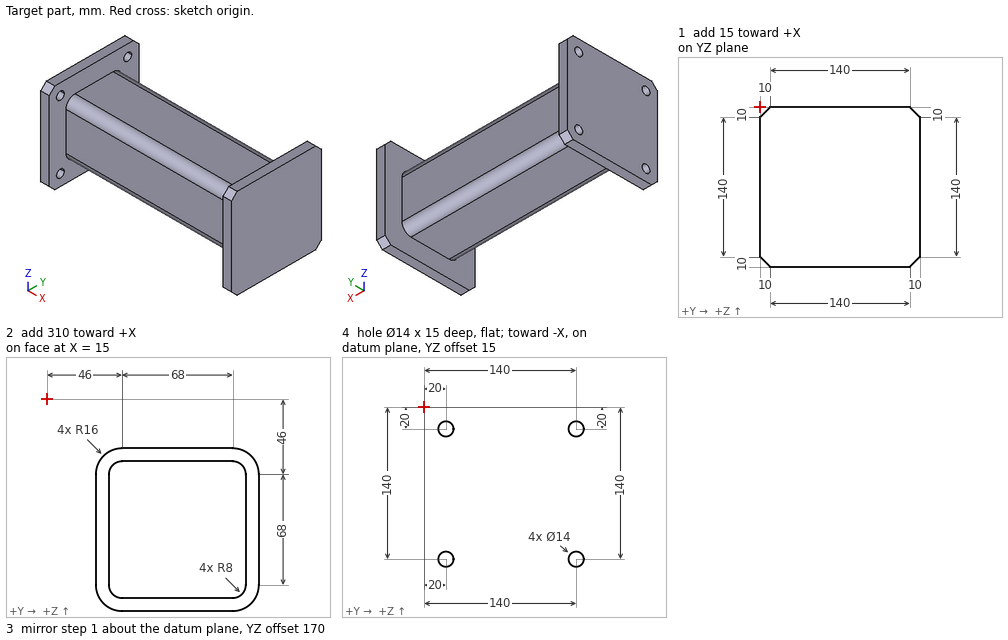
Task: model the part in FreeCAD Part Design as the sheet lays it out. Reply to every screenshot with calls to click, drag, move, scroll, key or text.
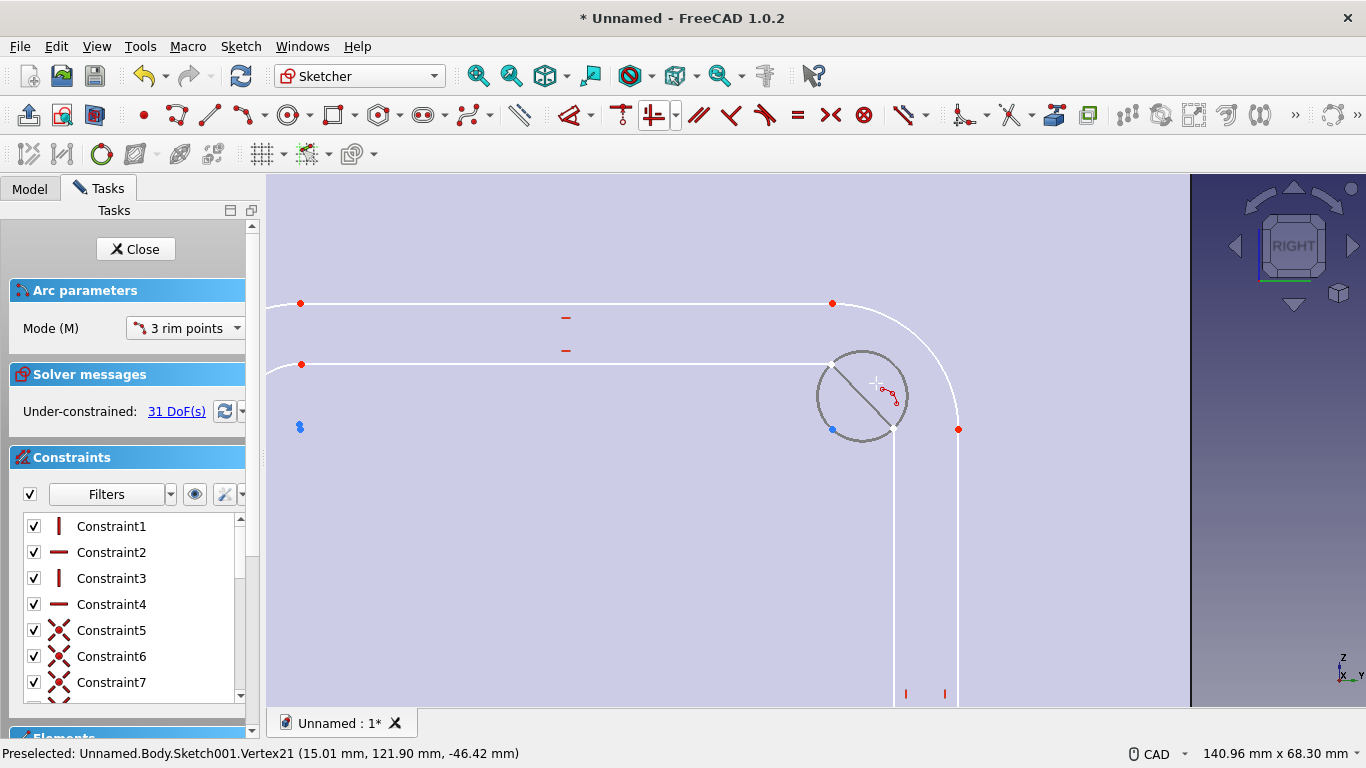
click(876, 381)
key(Escape)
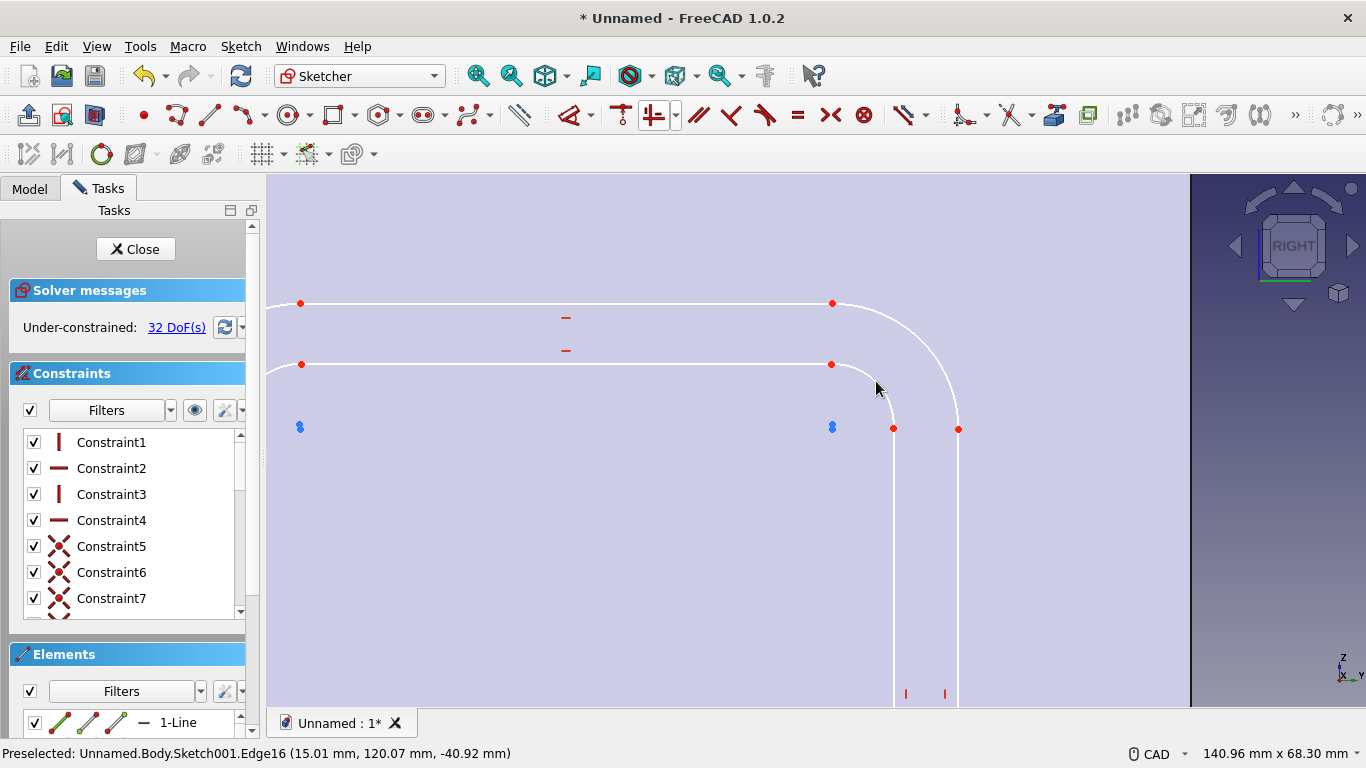
click(958, 588)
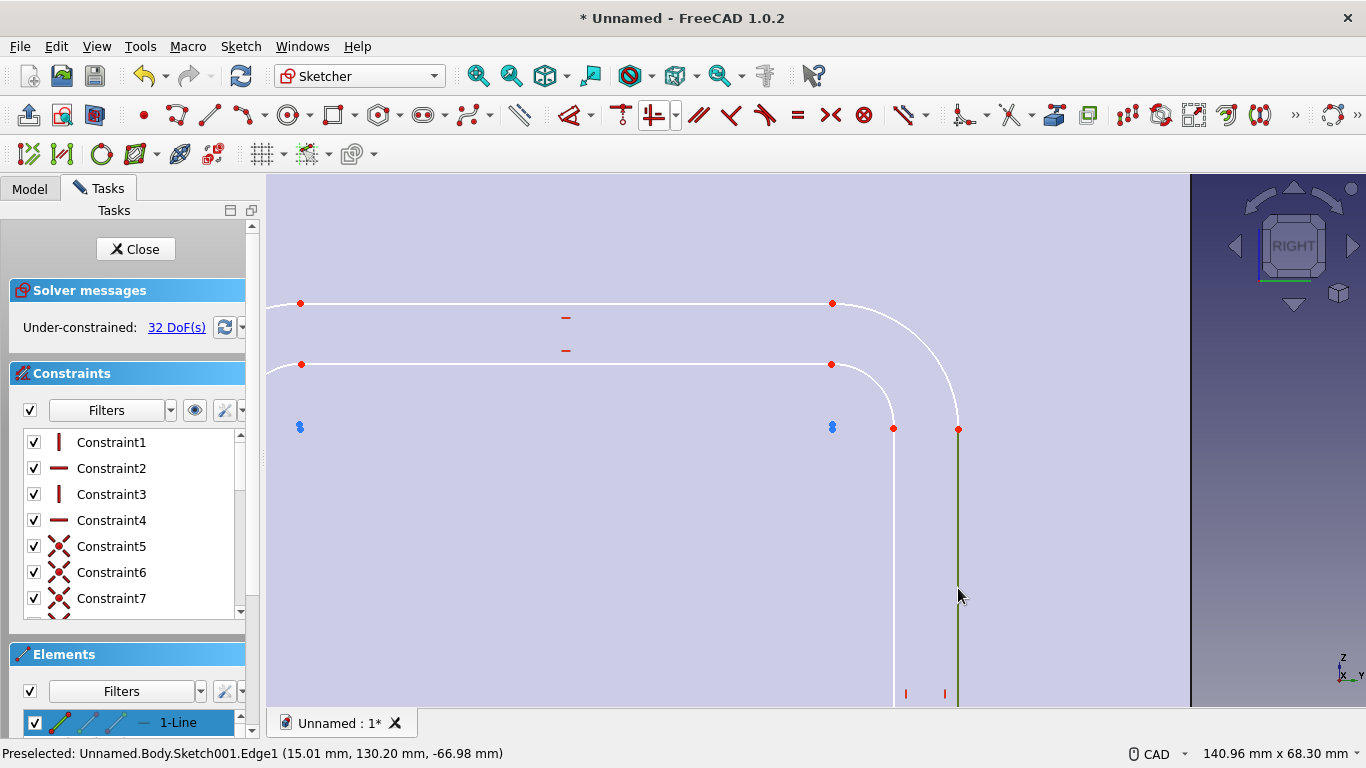
click(945, 373)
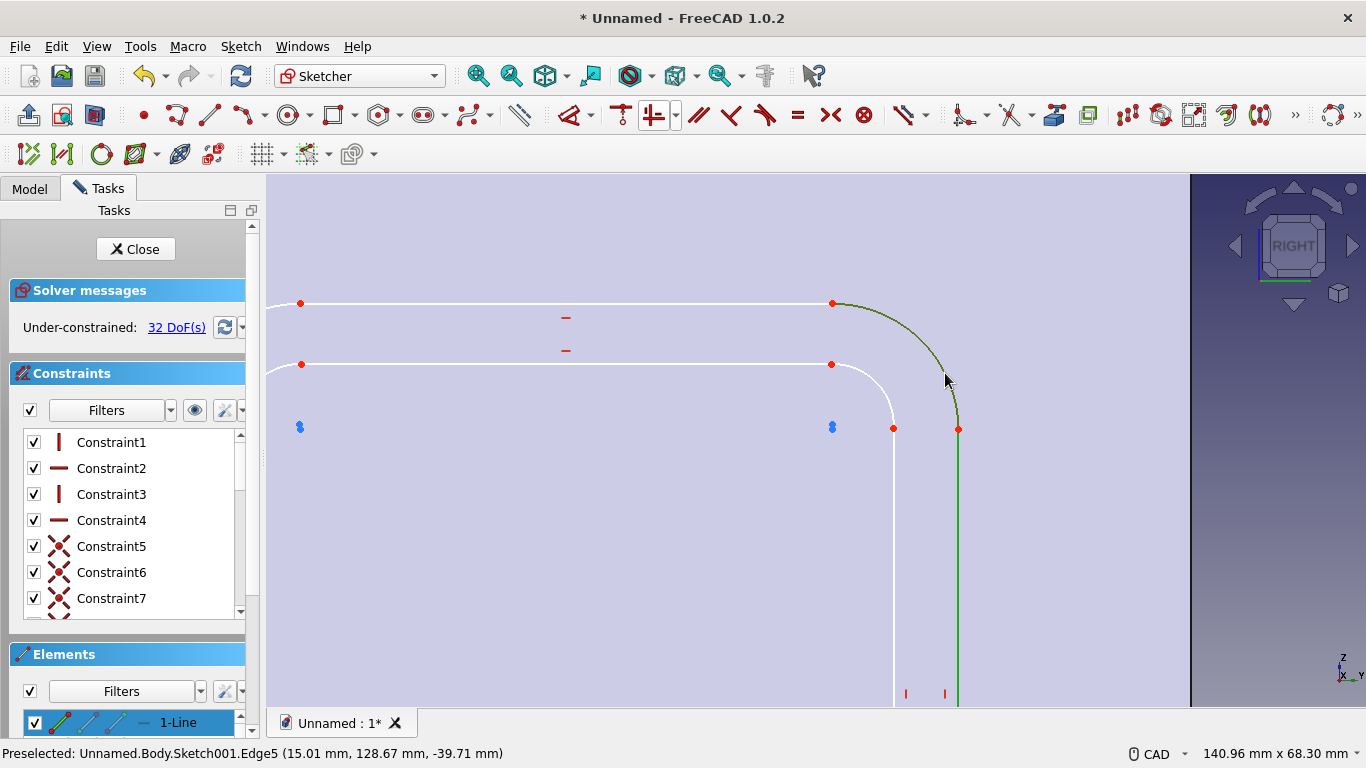
click(765, 116)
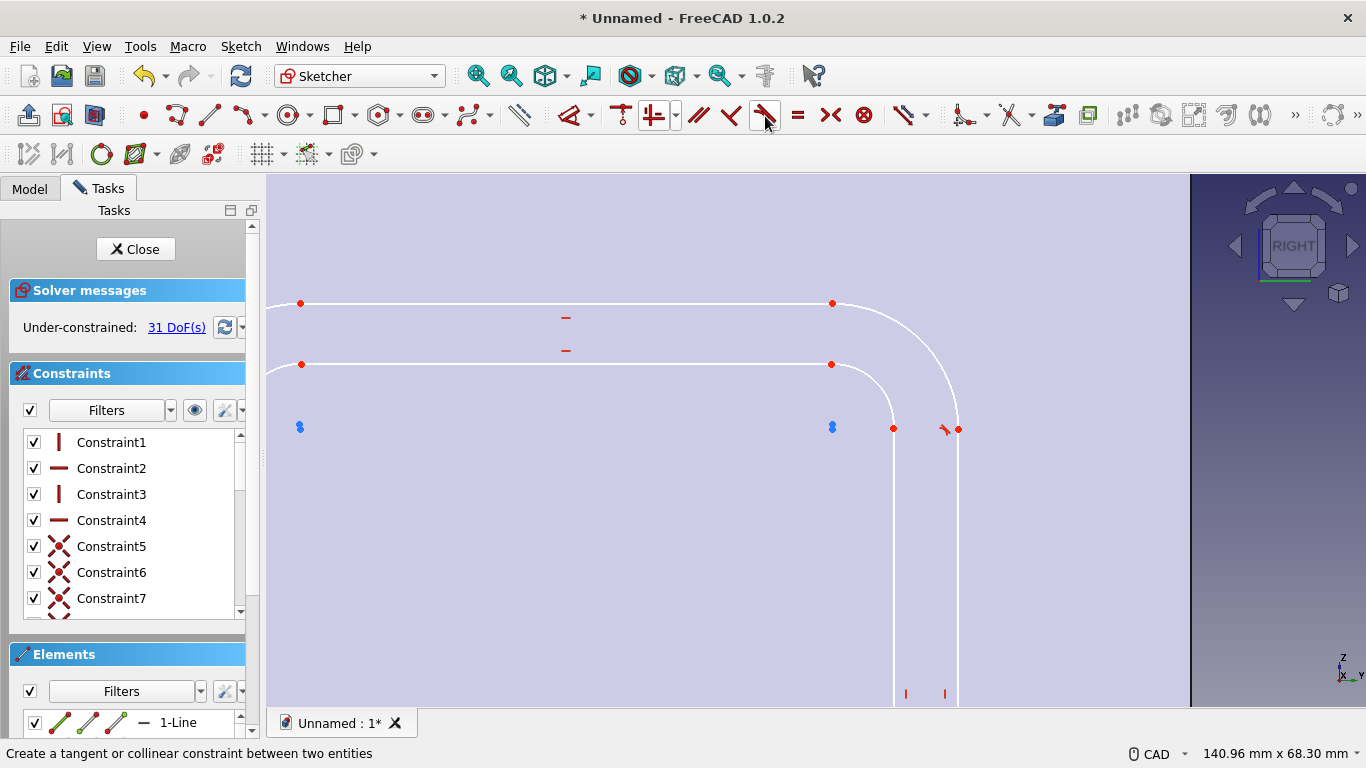
click(958, 588)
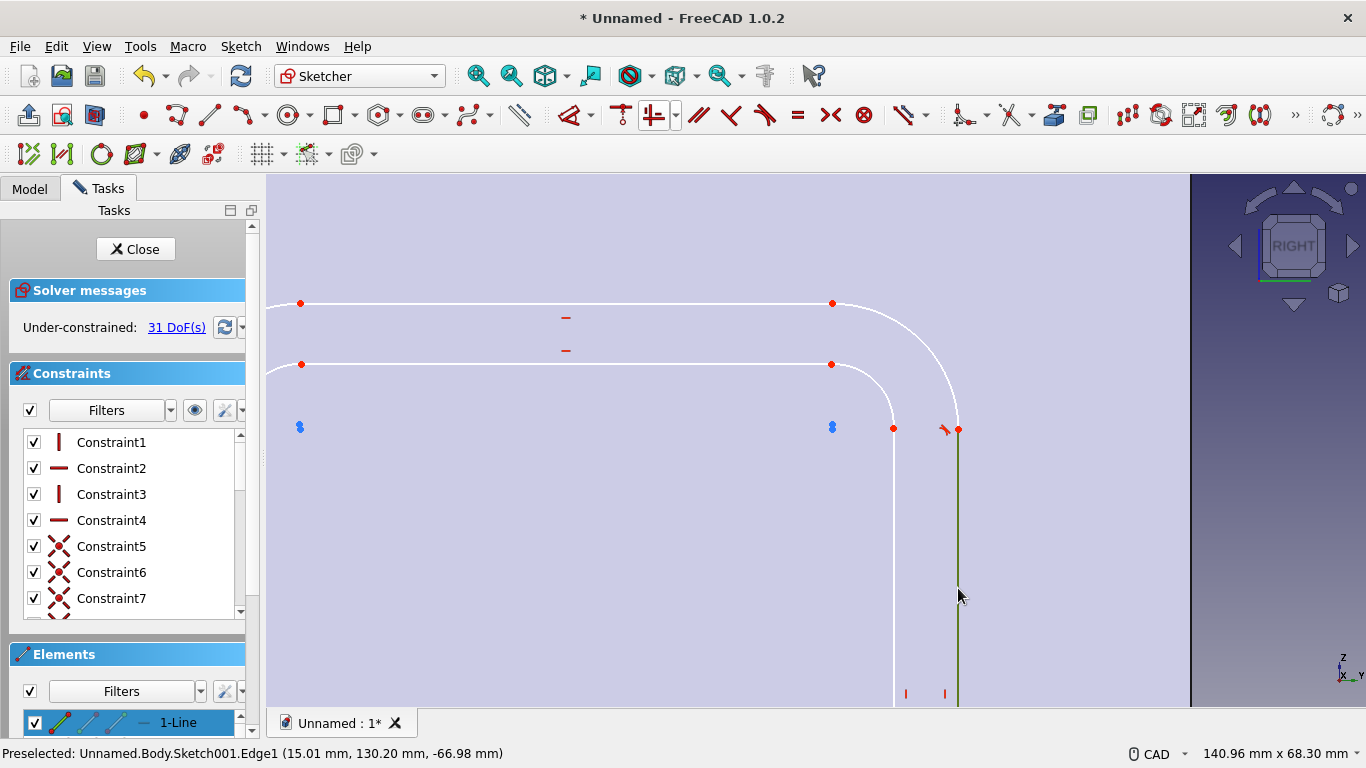
scroll(876, 383, down, 6)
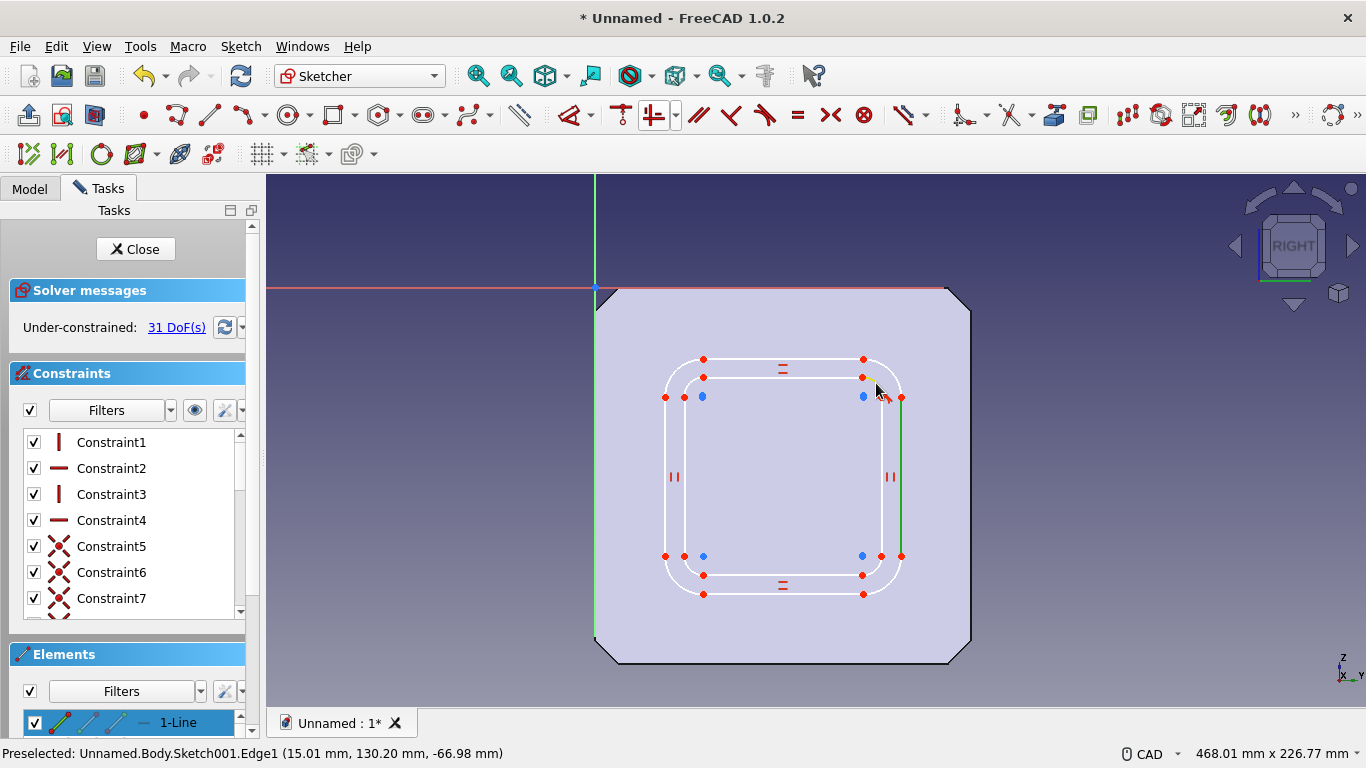
click(880, 590)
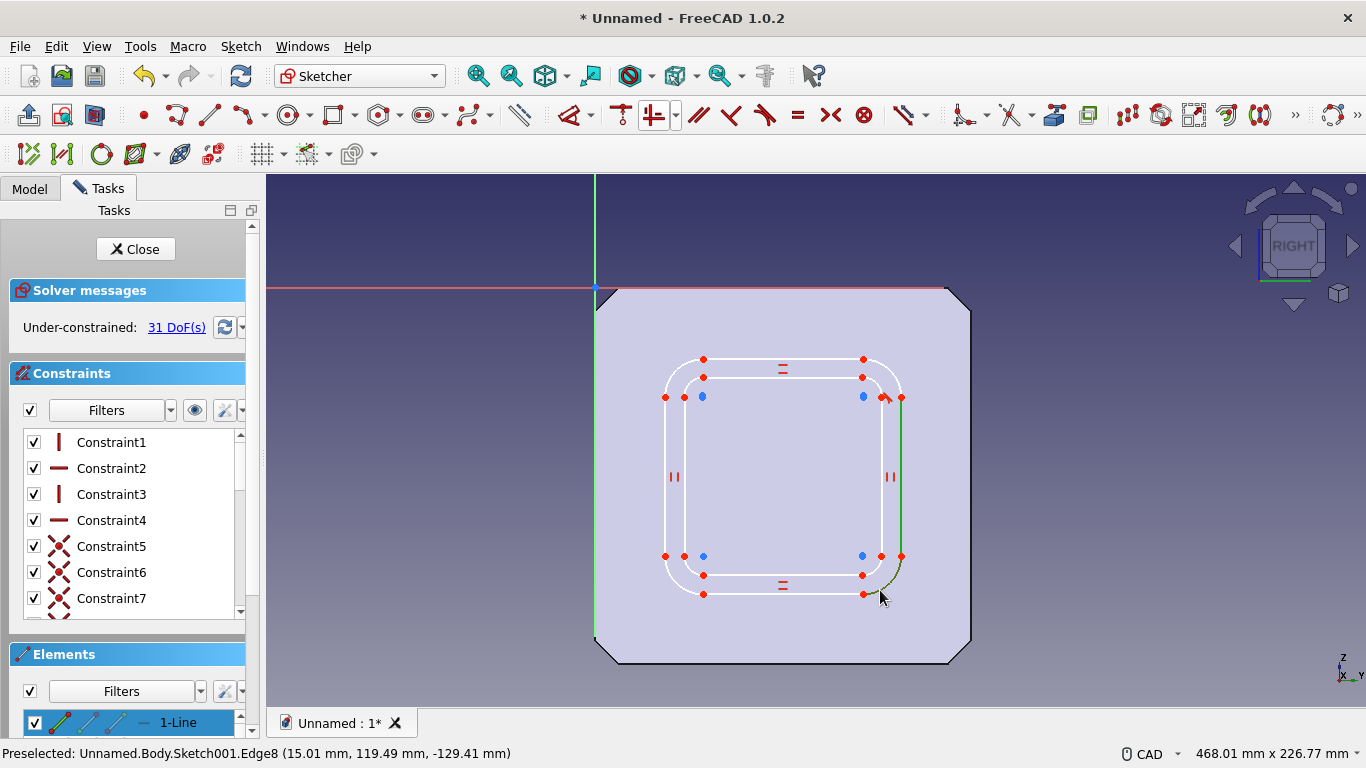
key(t)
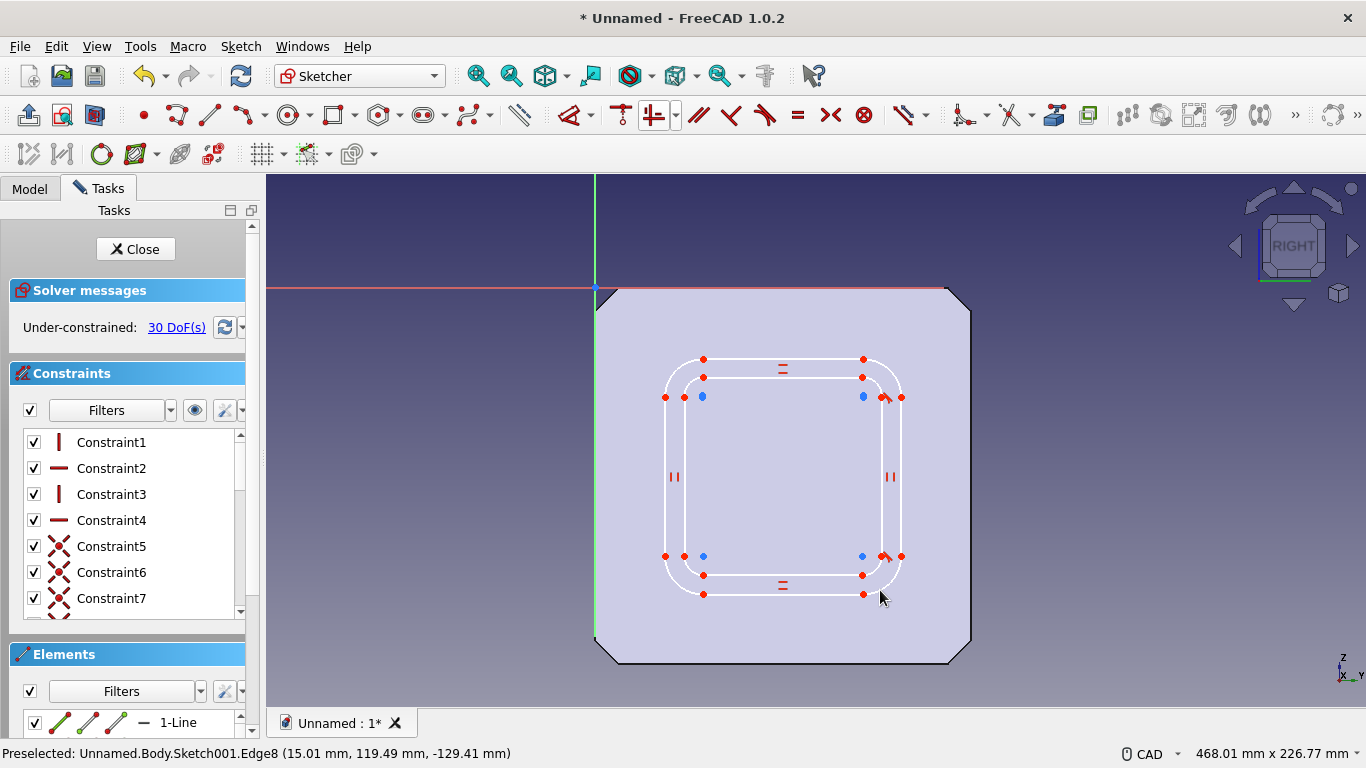
click(815, 359)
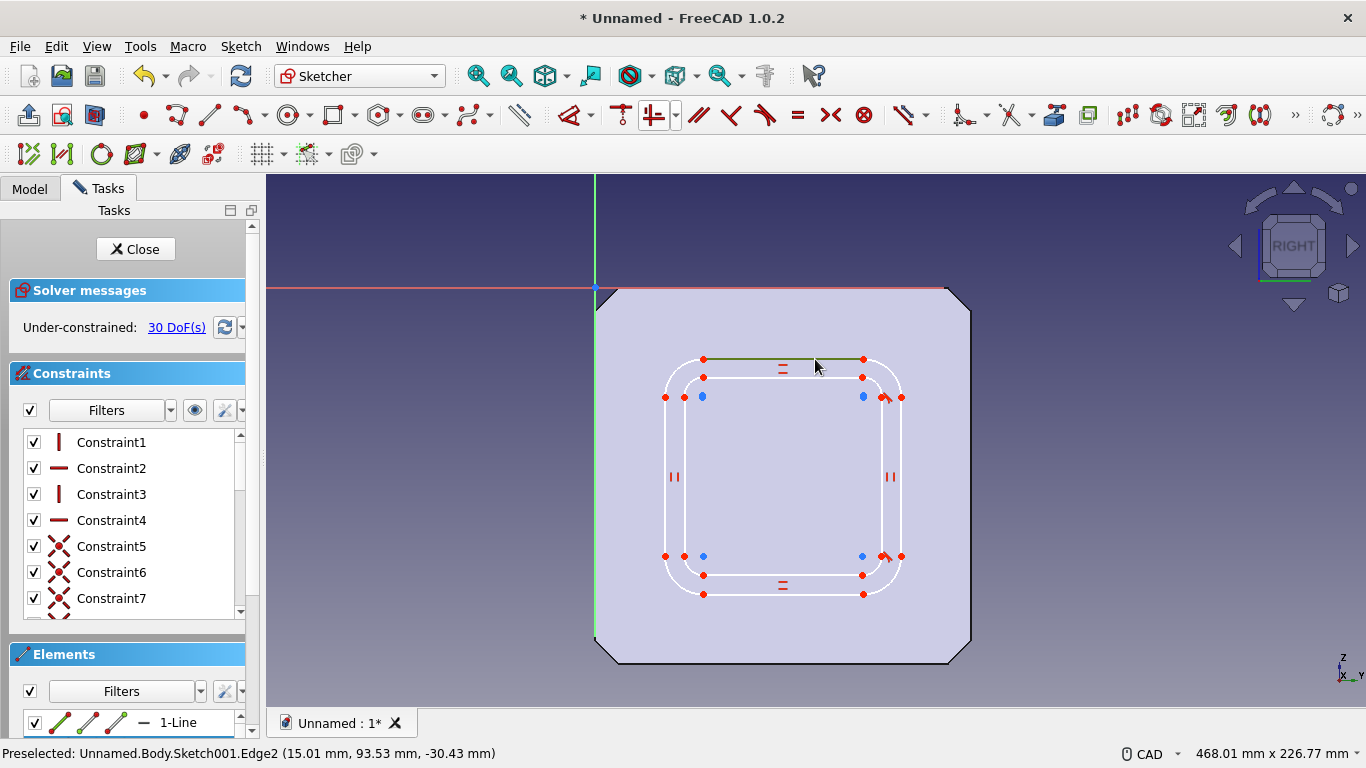
click(897, 380)